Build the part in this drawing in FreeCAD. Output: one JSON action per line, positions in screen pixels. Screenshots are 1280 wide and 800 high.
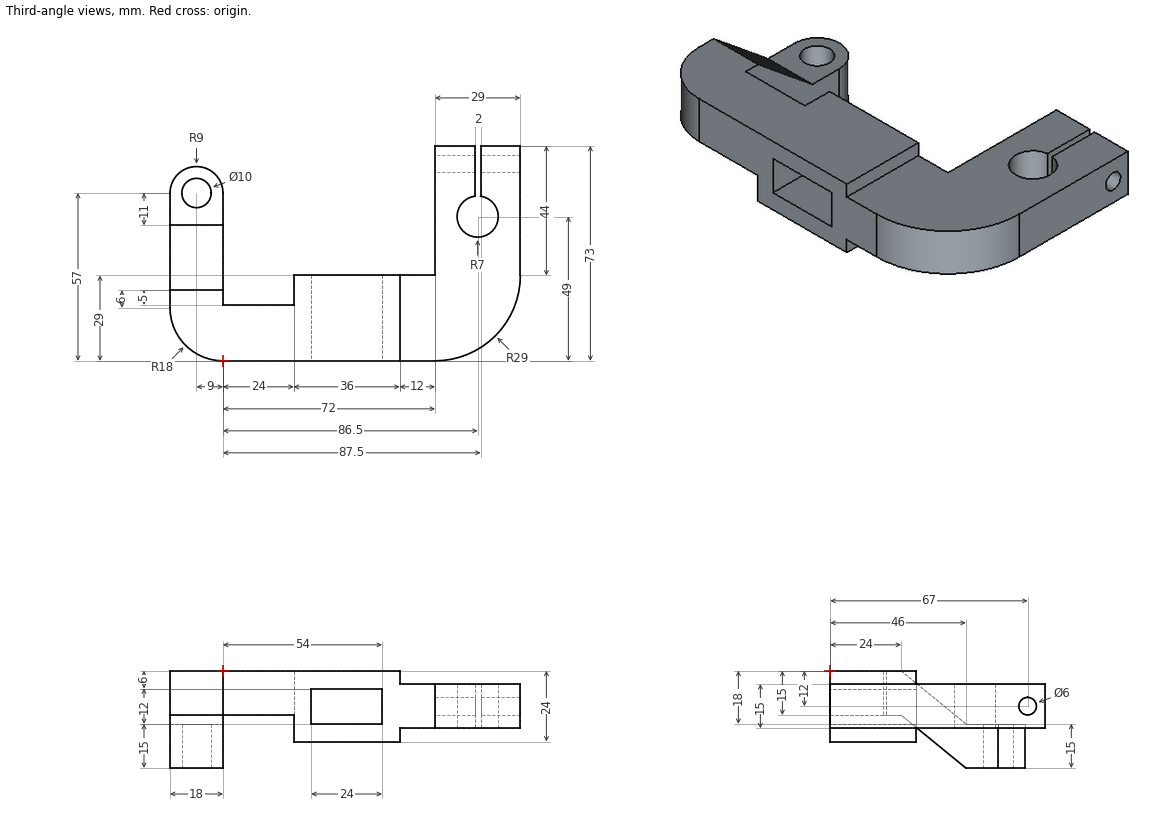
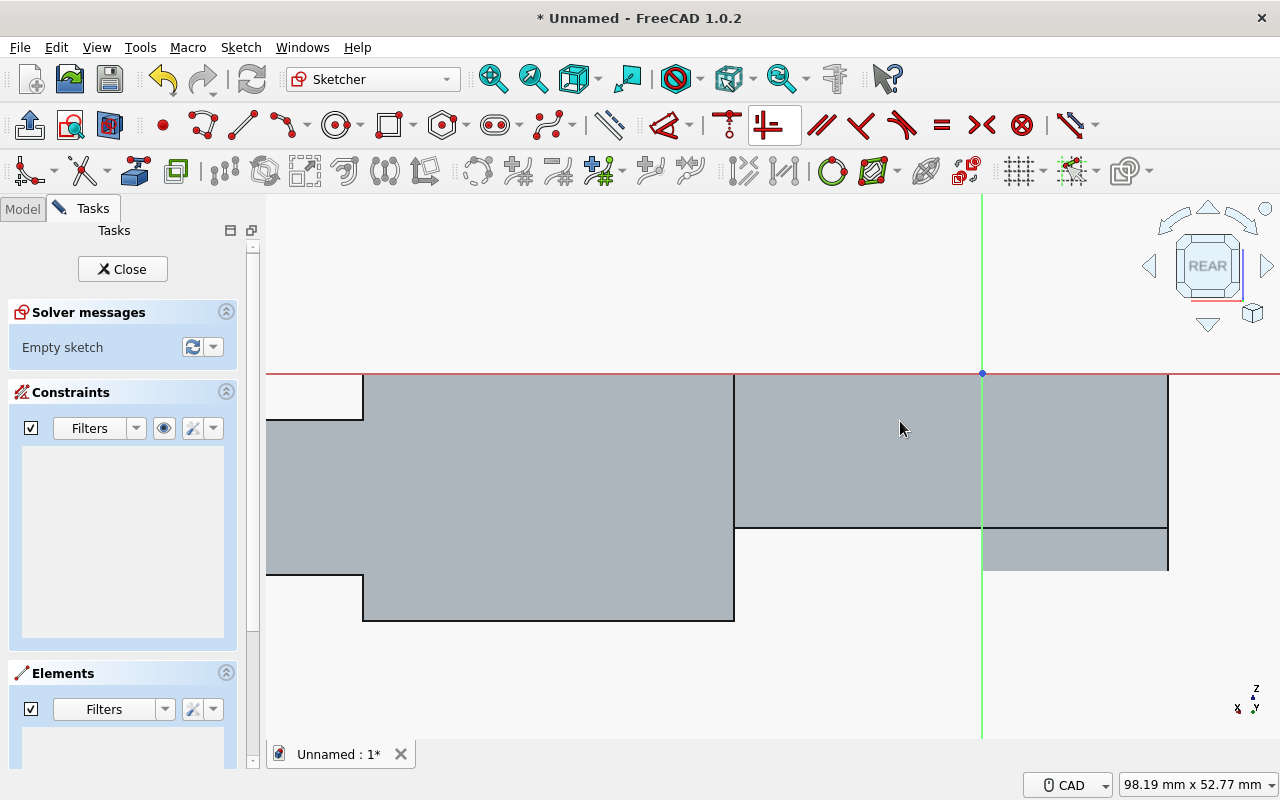
{"action": "left_click", "coordinate": [390, 126]}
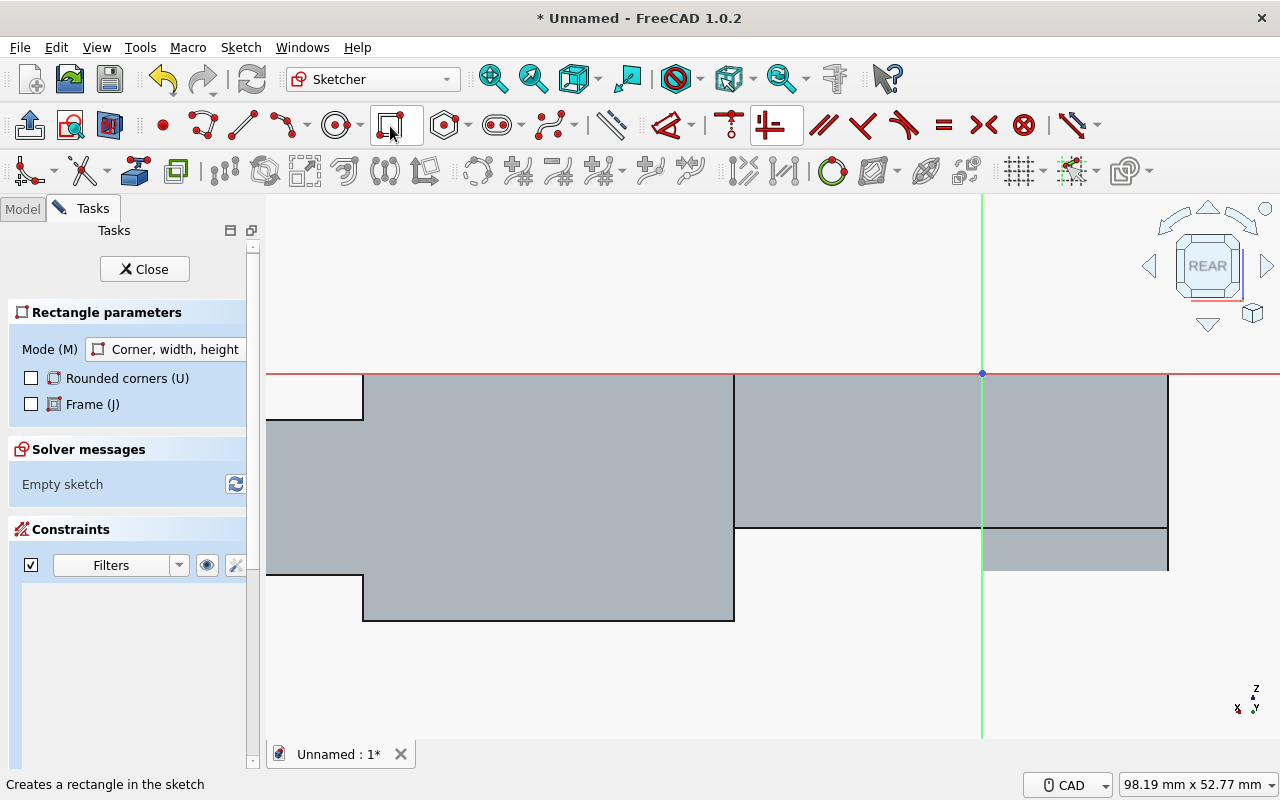
{"action": "left_click", "coordinate": [425, 436]}
{"action": "mouse_move", "coordinate": [672, 559]}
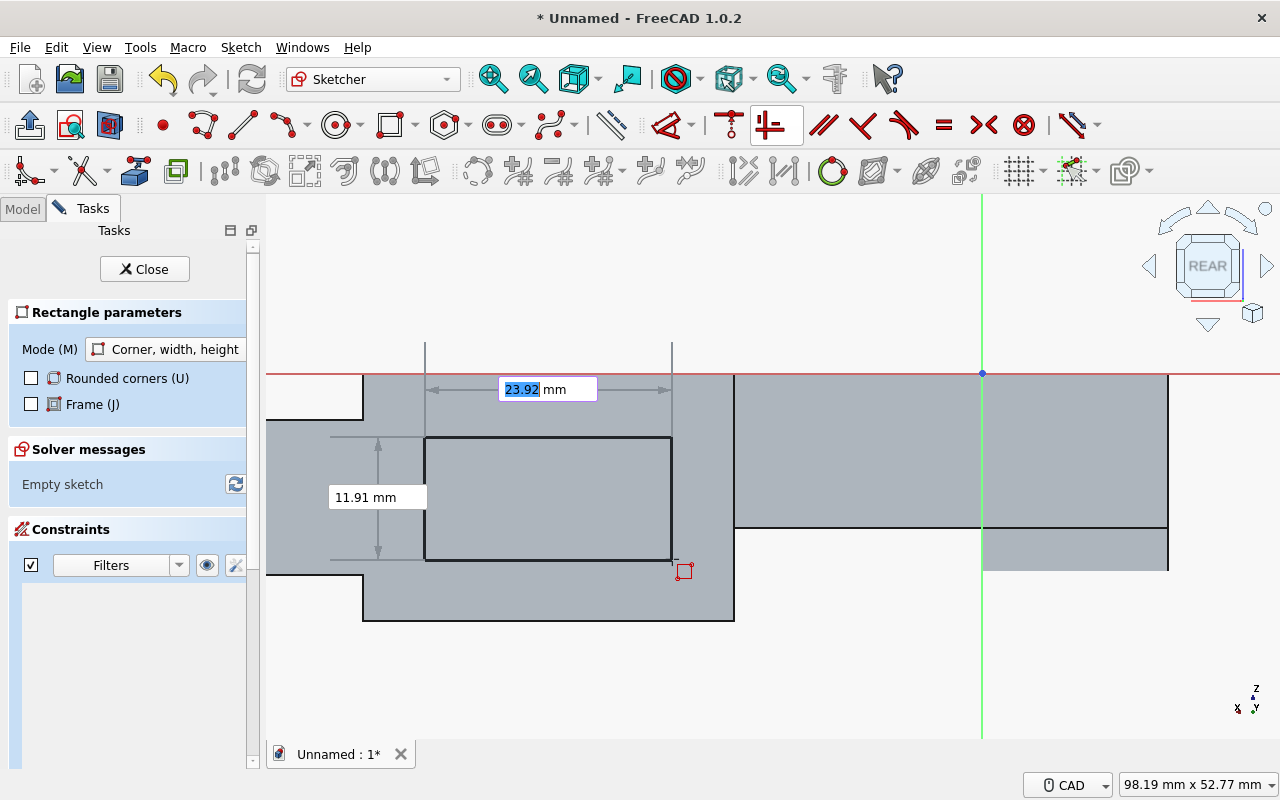
{"action": "type", "text": "24"}
{"action": "key", "text": "Tab"}
{"action": "type", "text": "12"}
{"action": "key", "text": "Return"}
{"action": "key", "text": "Escape"}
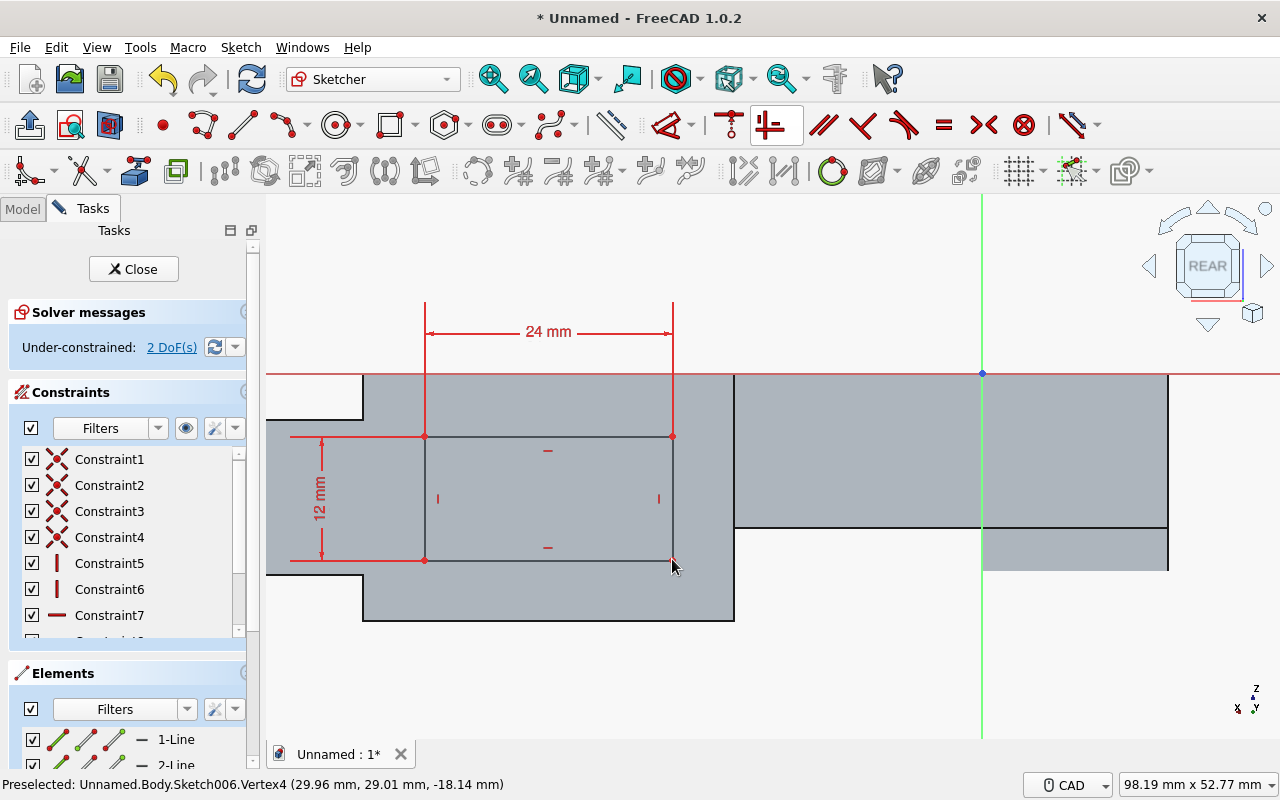
{"action": "left_click", "coordinate": [666, 126]}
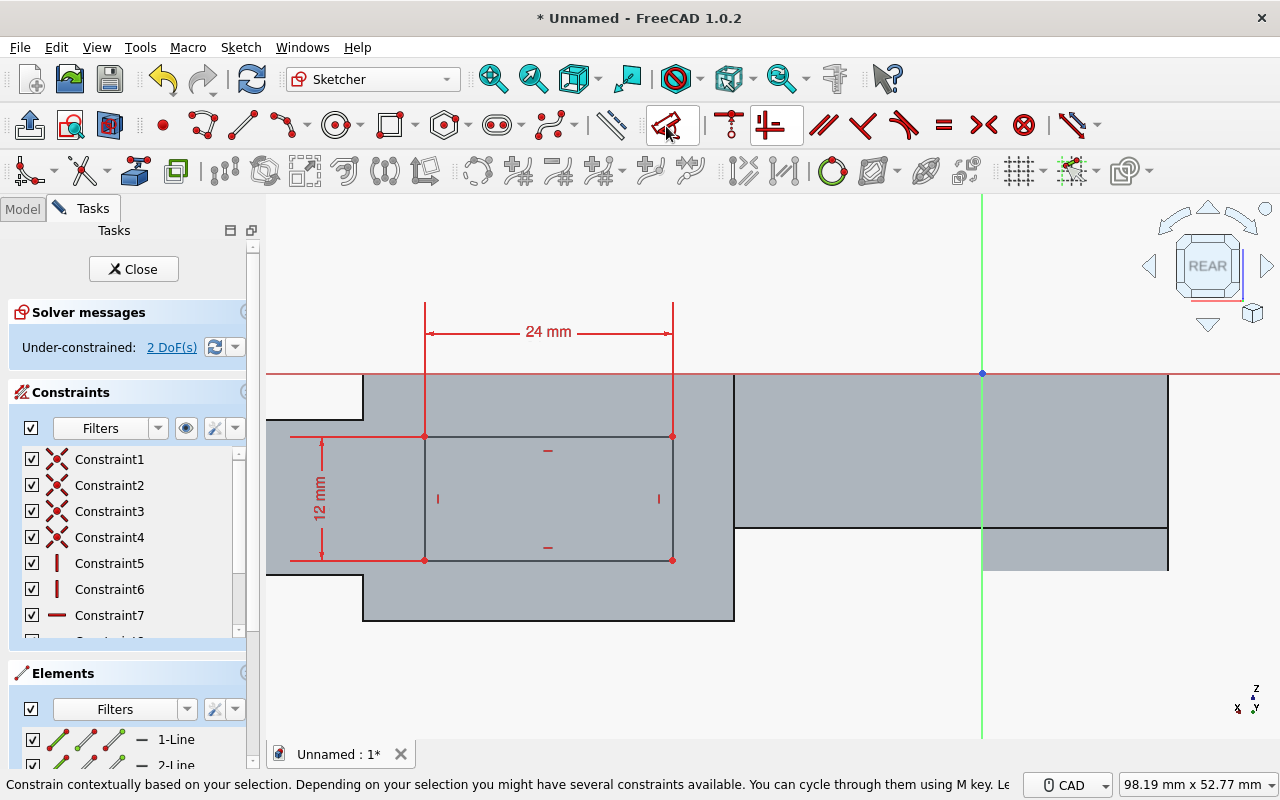
{"action": "left_click", "coordinate": [425, 437]}
{"action": "left_click", "coordinate": [1016, 405]}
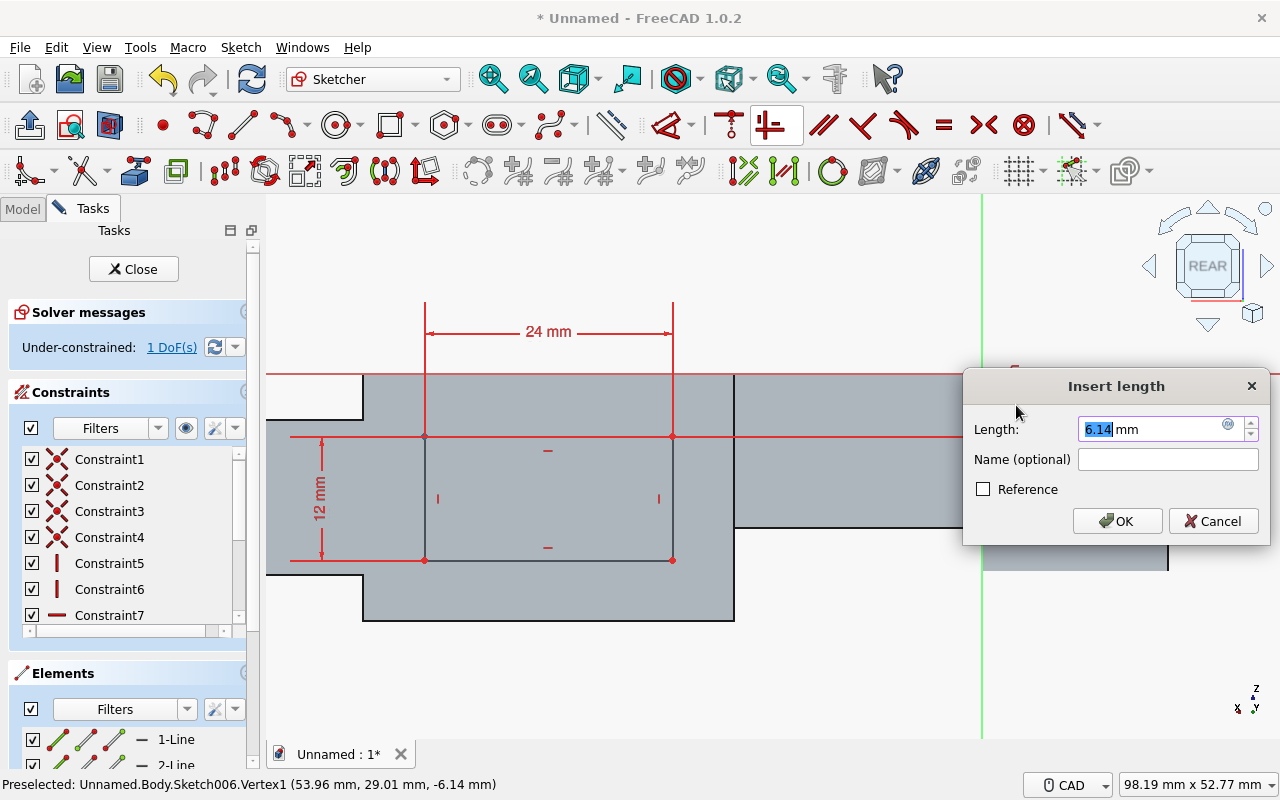
{"action": "type", "text": "6"}
{"action": "key", "text": "Return"}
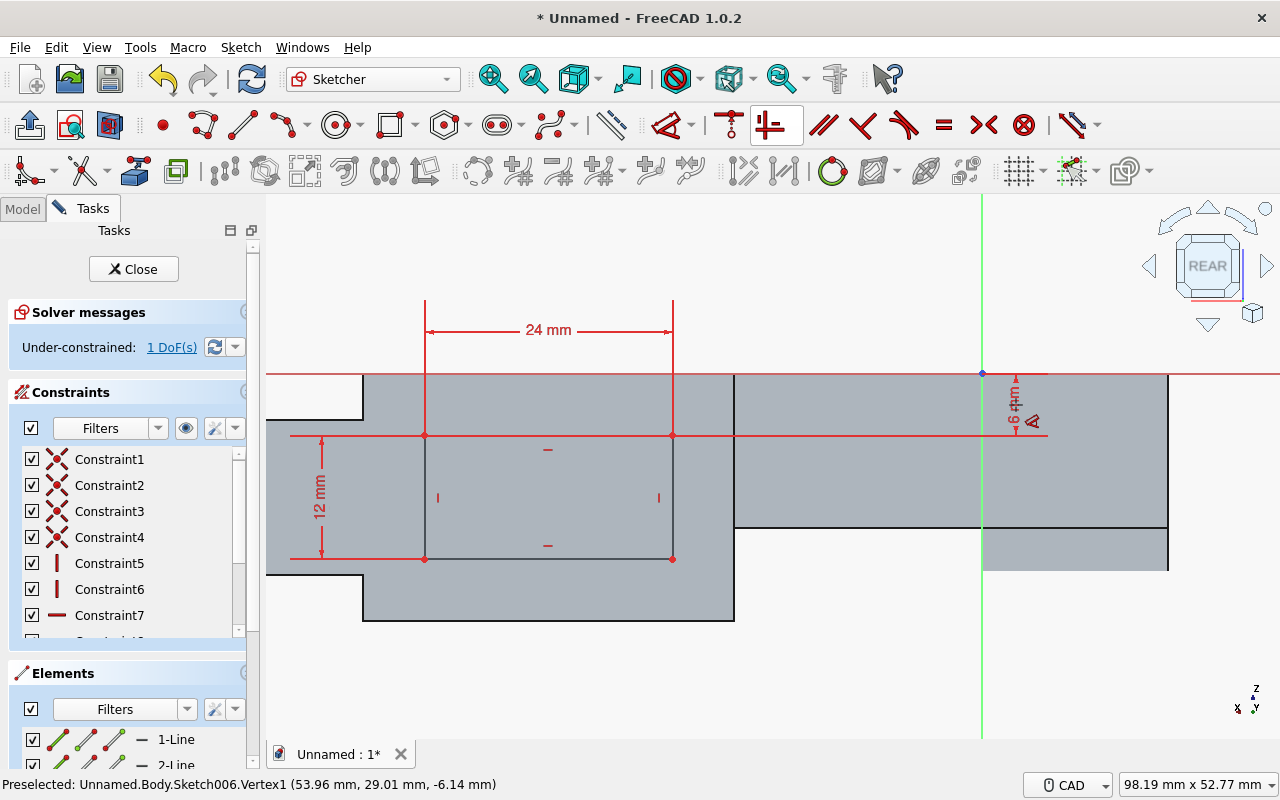
{"action": "left_click", "coordinate": [425, 436]}
{"action": "left_click", "coordinate": [704, 340]}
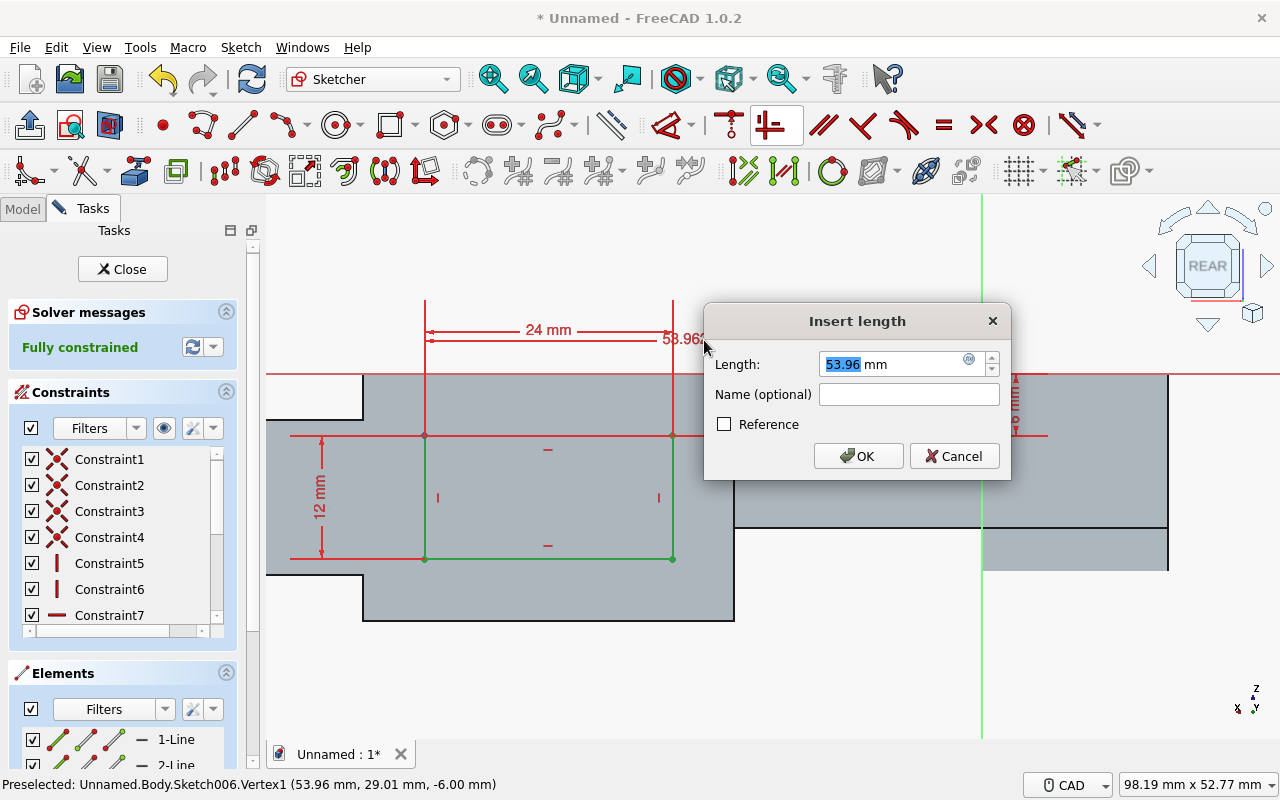
{"action": "type", "text": "54"}
{"action": "key", "text": "Return"}
{"action": "key", "text": "Escape"}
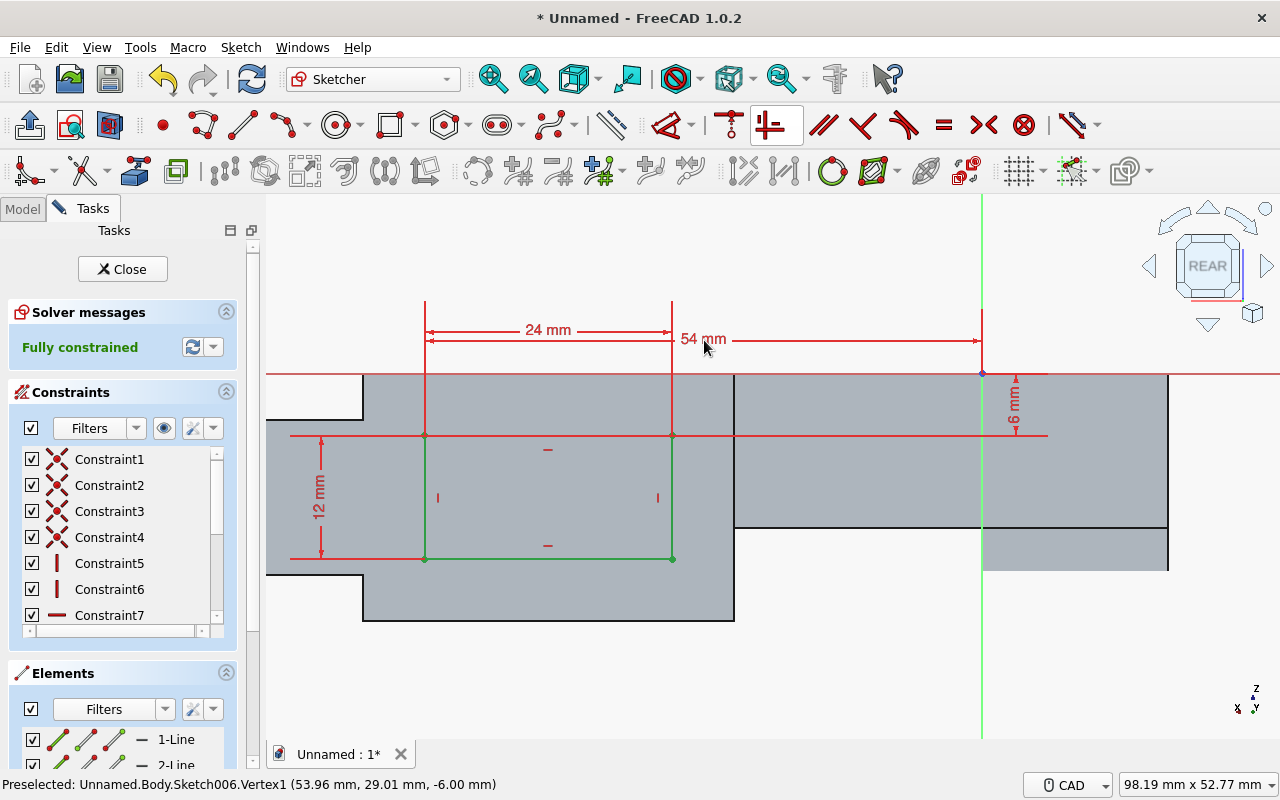
{"action": "left_click", "coordinate": [123, 269]}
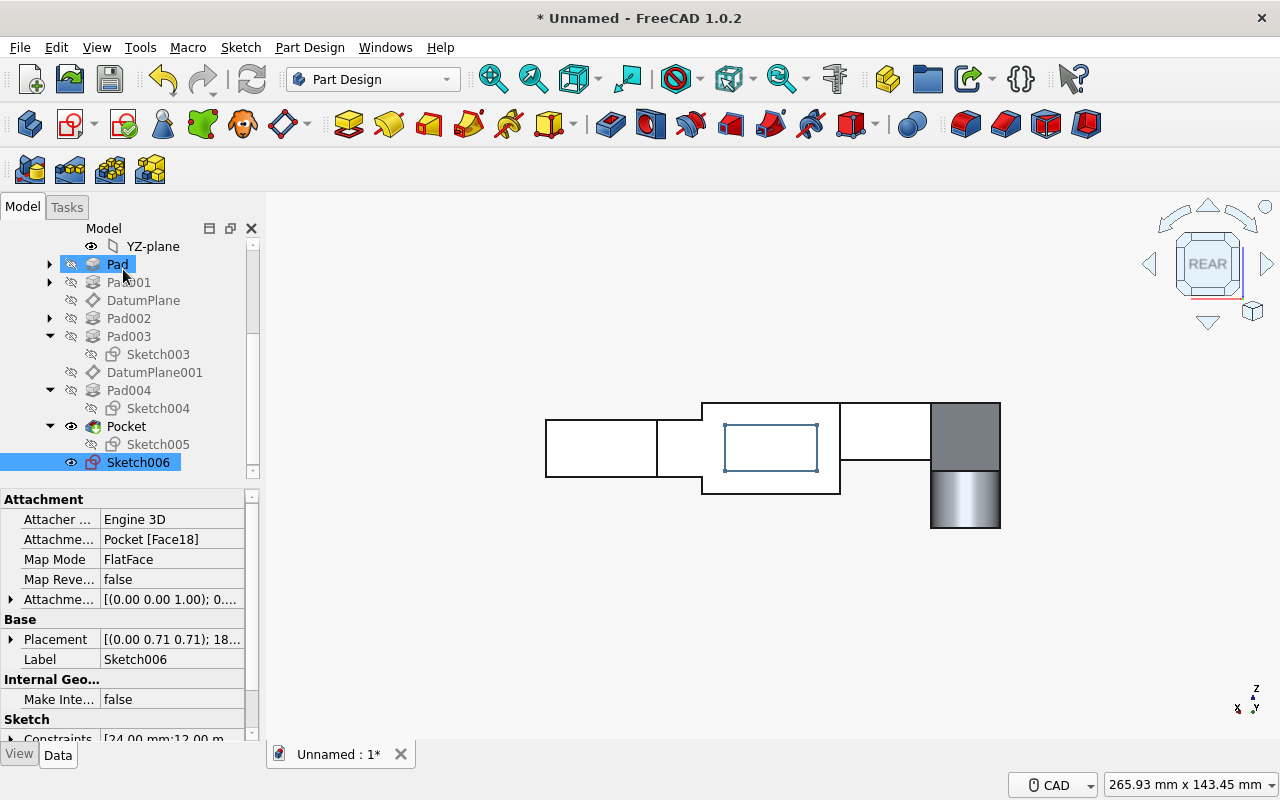
{"action": "left_click", "coordinate": [612, 124]}